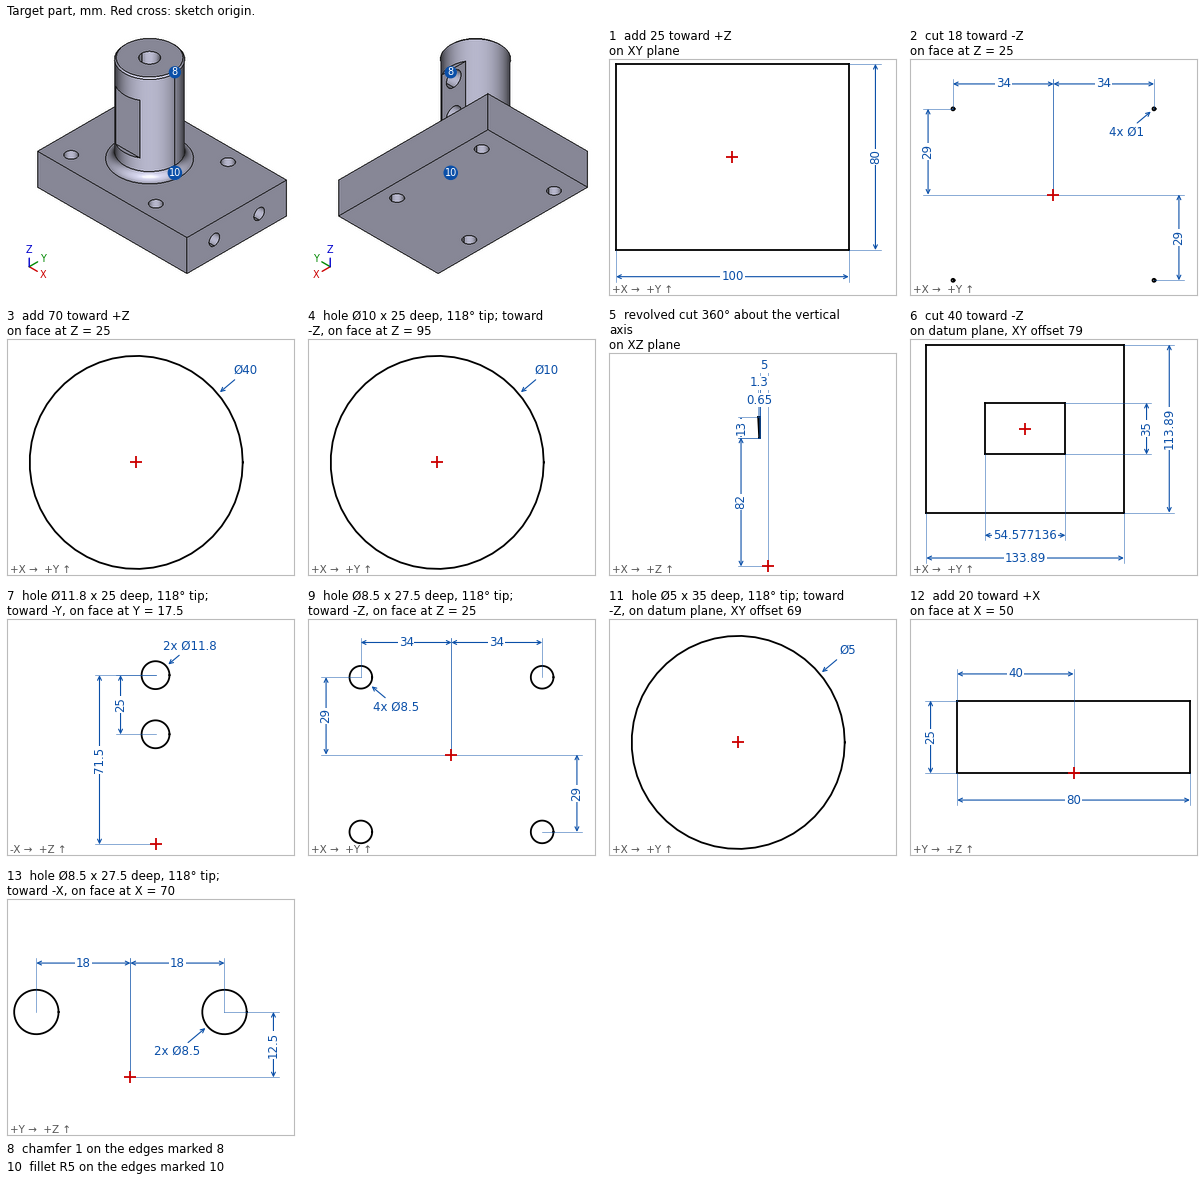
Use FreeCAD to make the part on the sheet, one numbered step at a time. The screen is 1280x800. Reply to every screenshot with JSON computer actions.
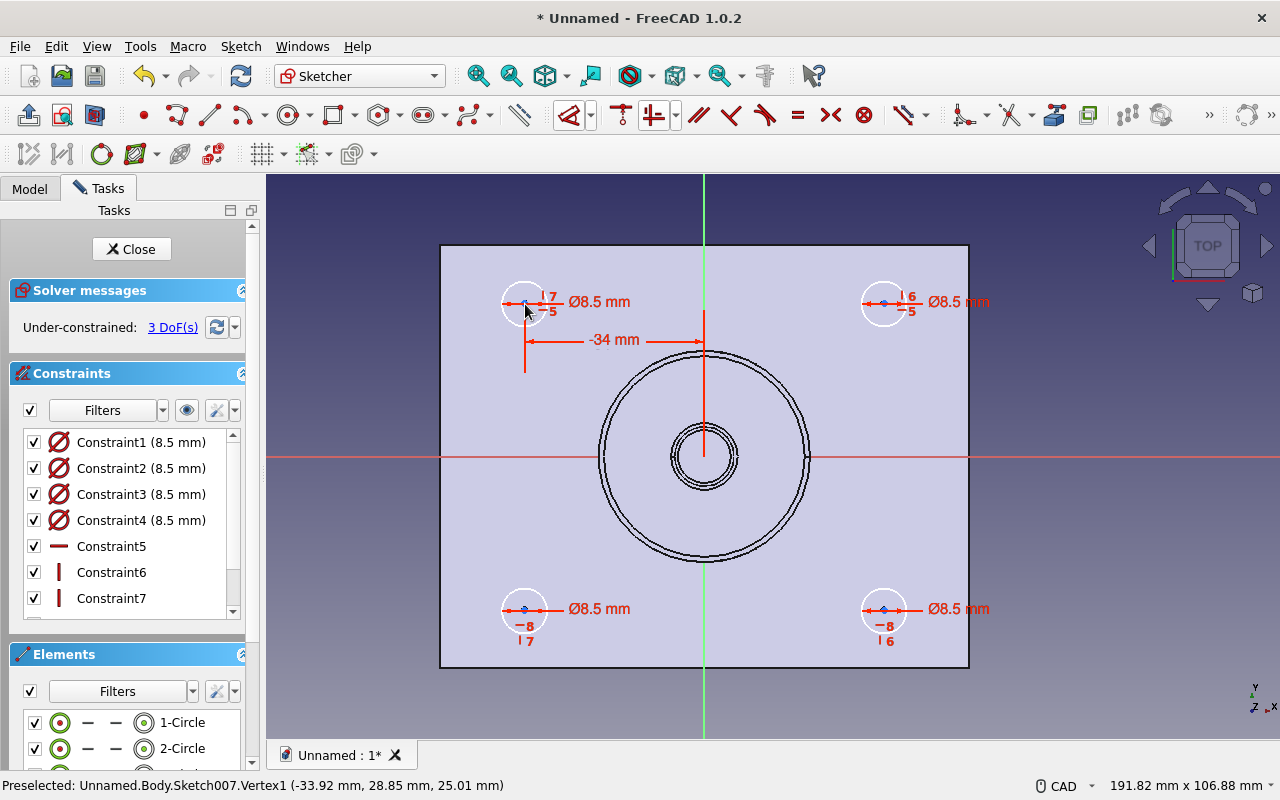
{"action": "left_click", "coordinate": [525, 304]}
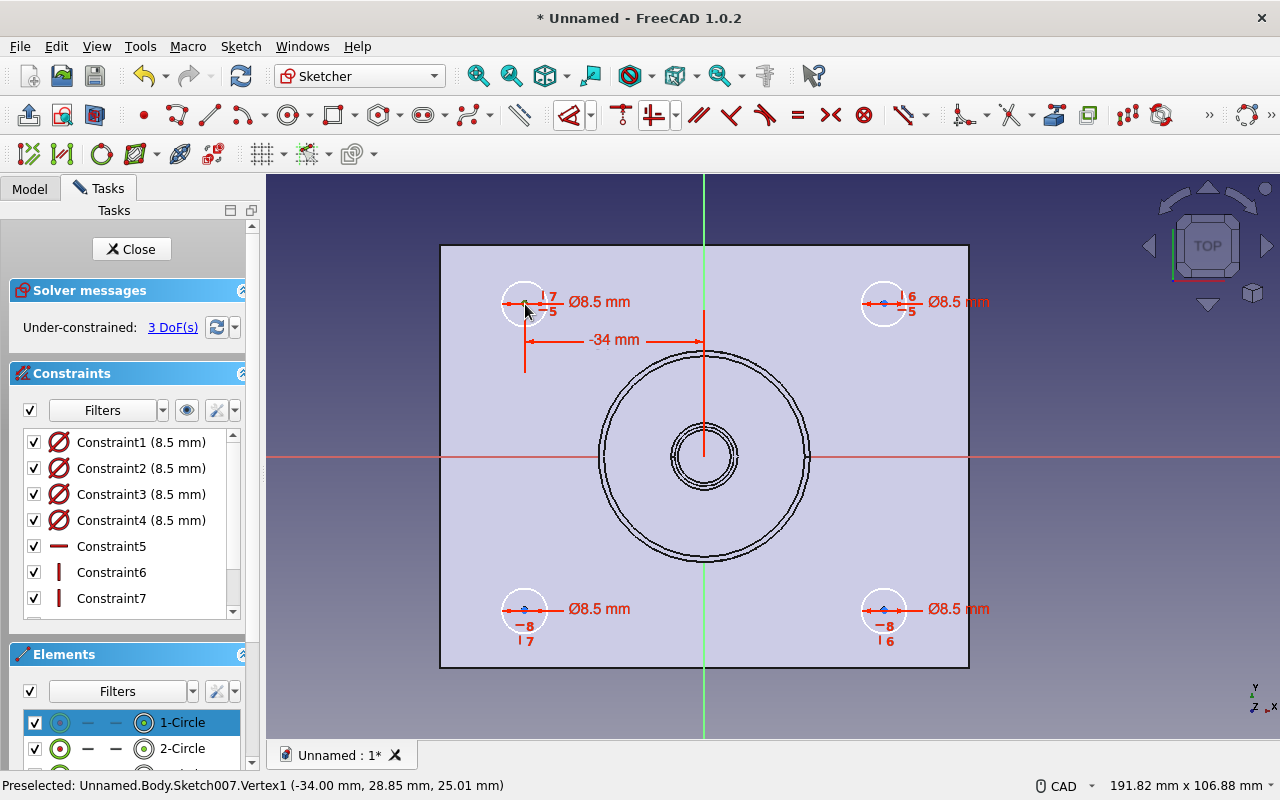
{"action": "key", "text": "i"}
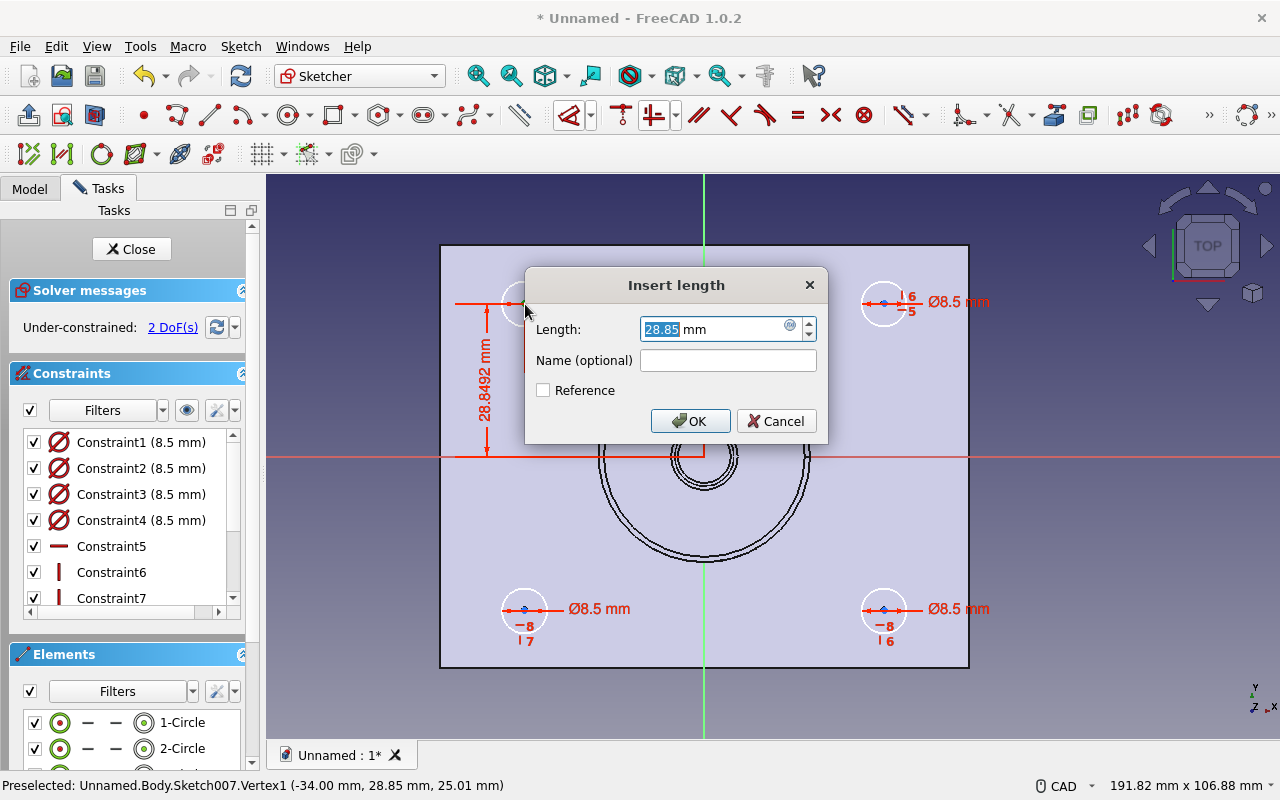
{"action": "type", "text": "29"}
{"action": "key", "text": "Return"}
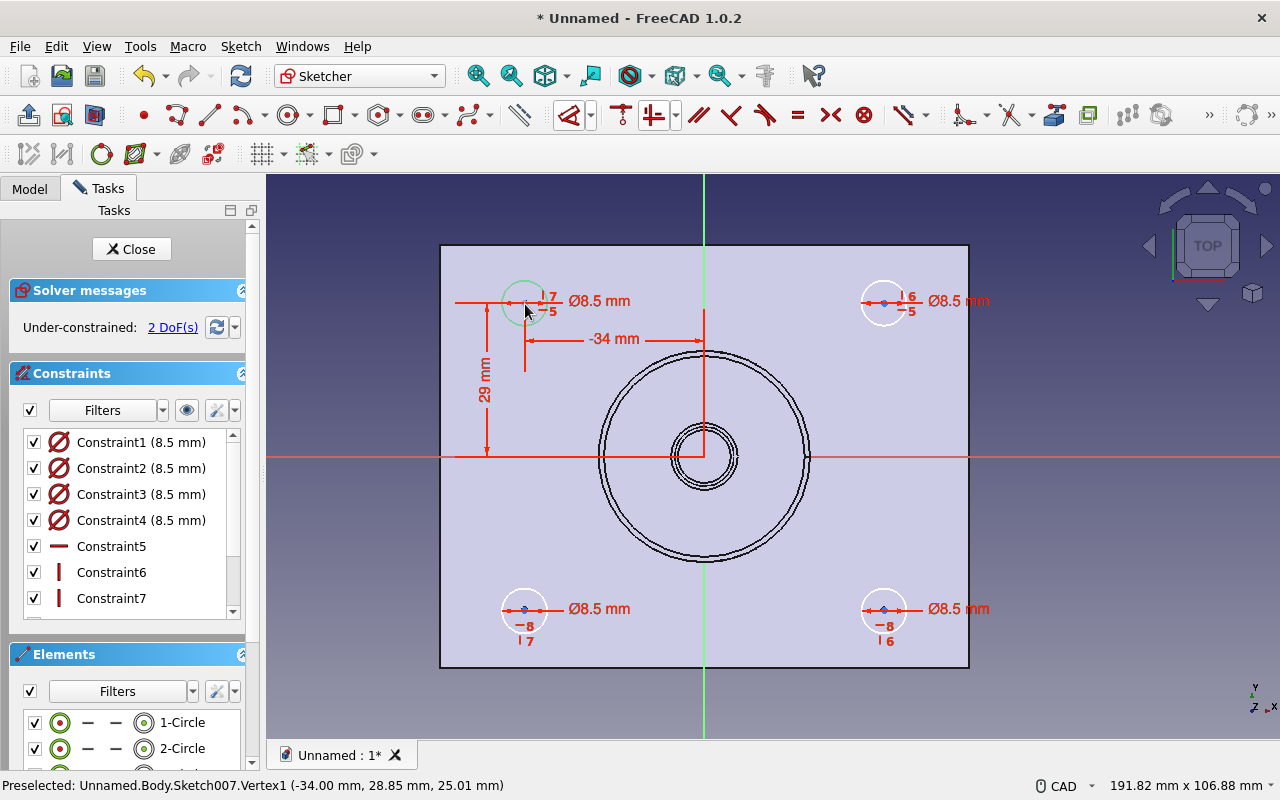
{"action": "left_click", "coordinate": [884, 303]}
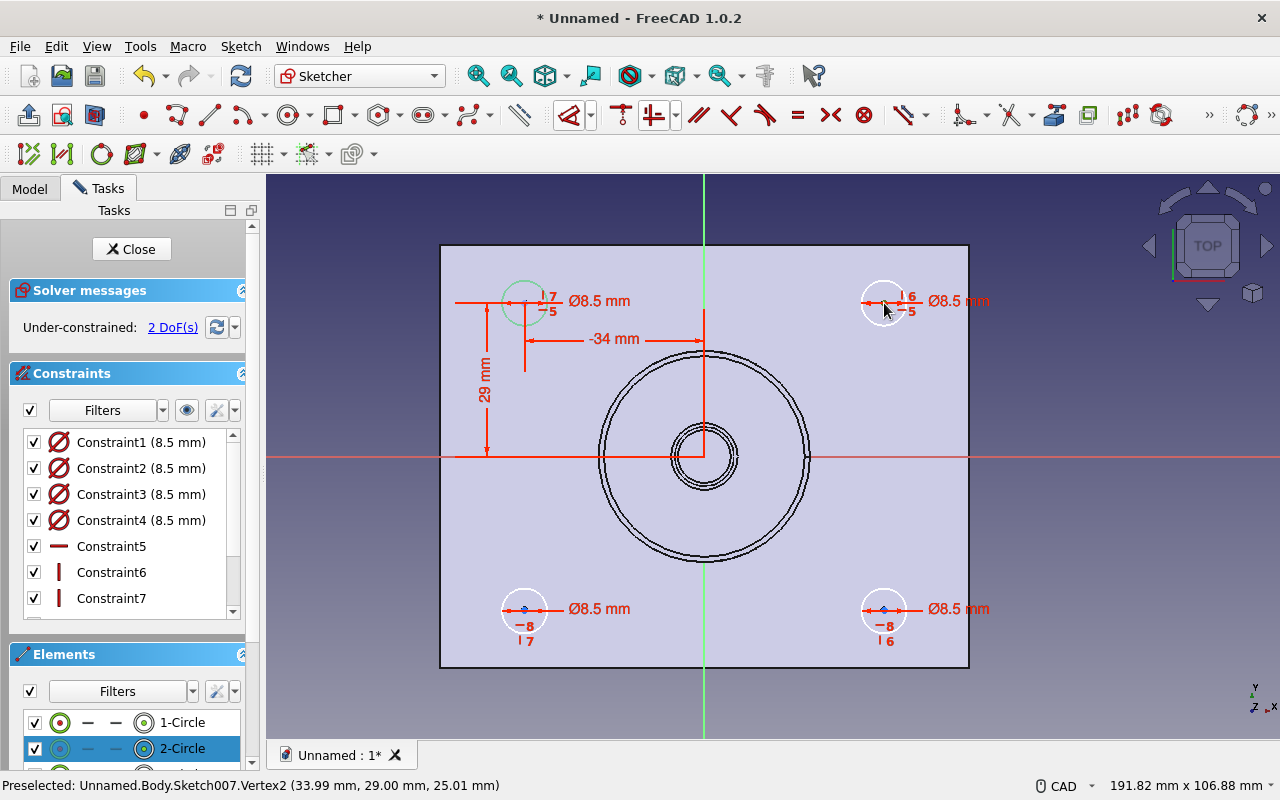
{"action": "key", "text": "l"}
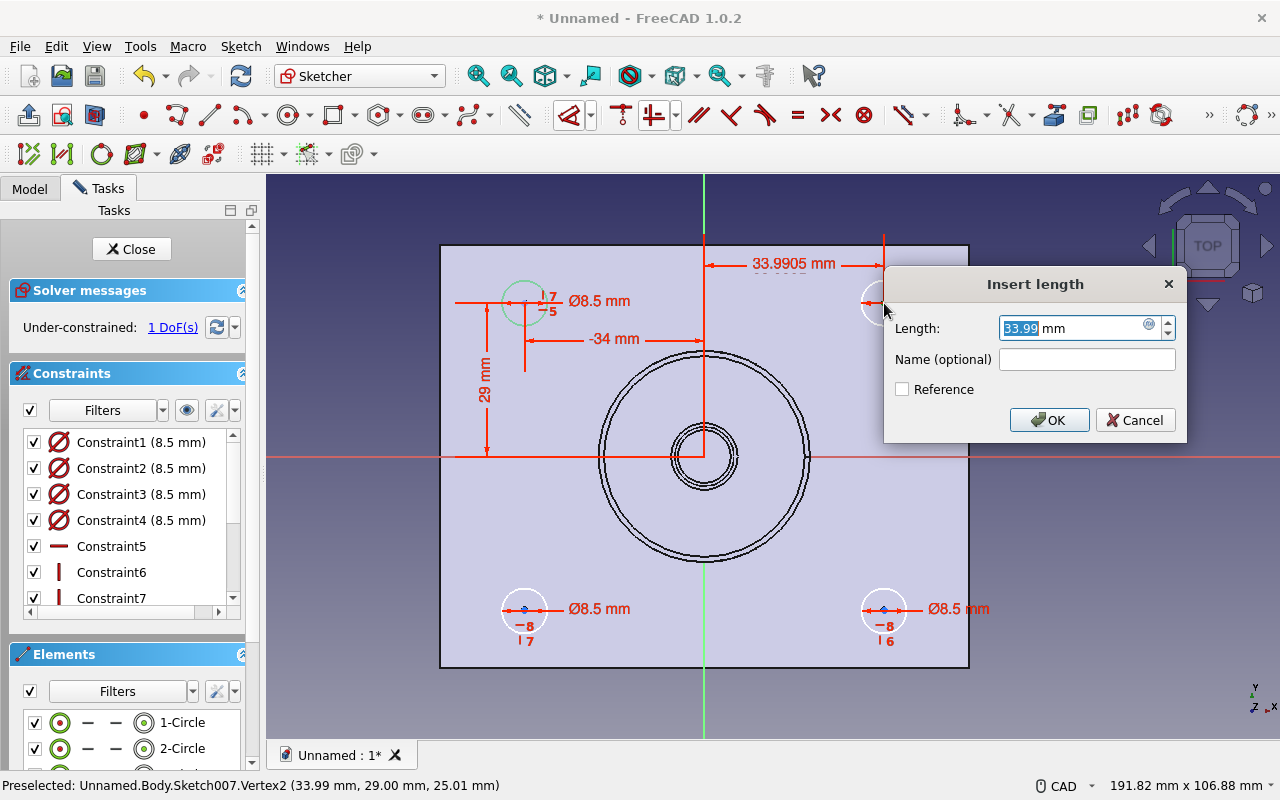
{"action": "type", "text": "34"}
{"action": "key", "text": "Return"}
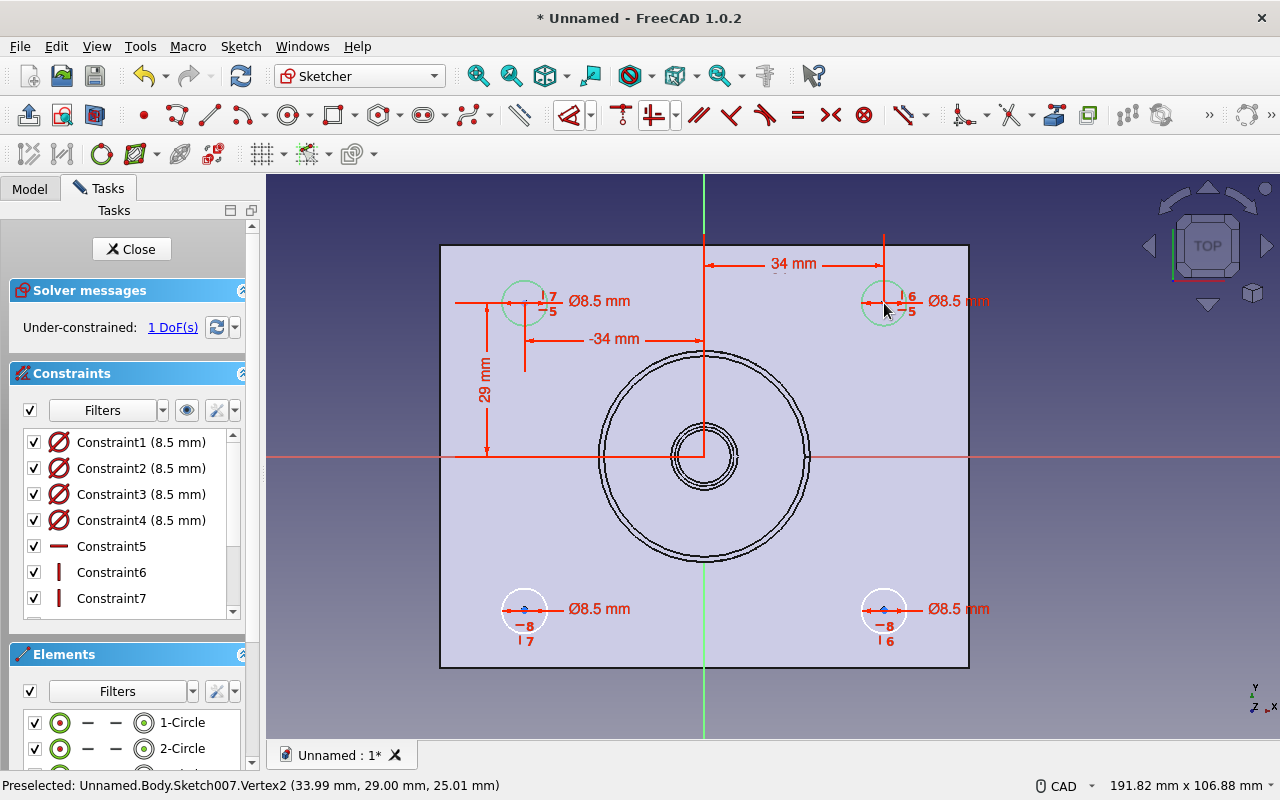
{"action": "left_click", "coordinate": [884, 611]}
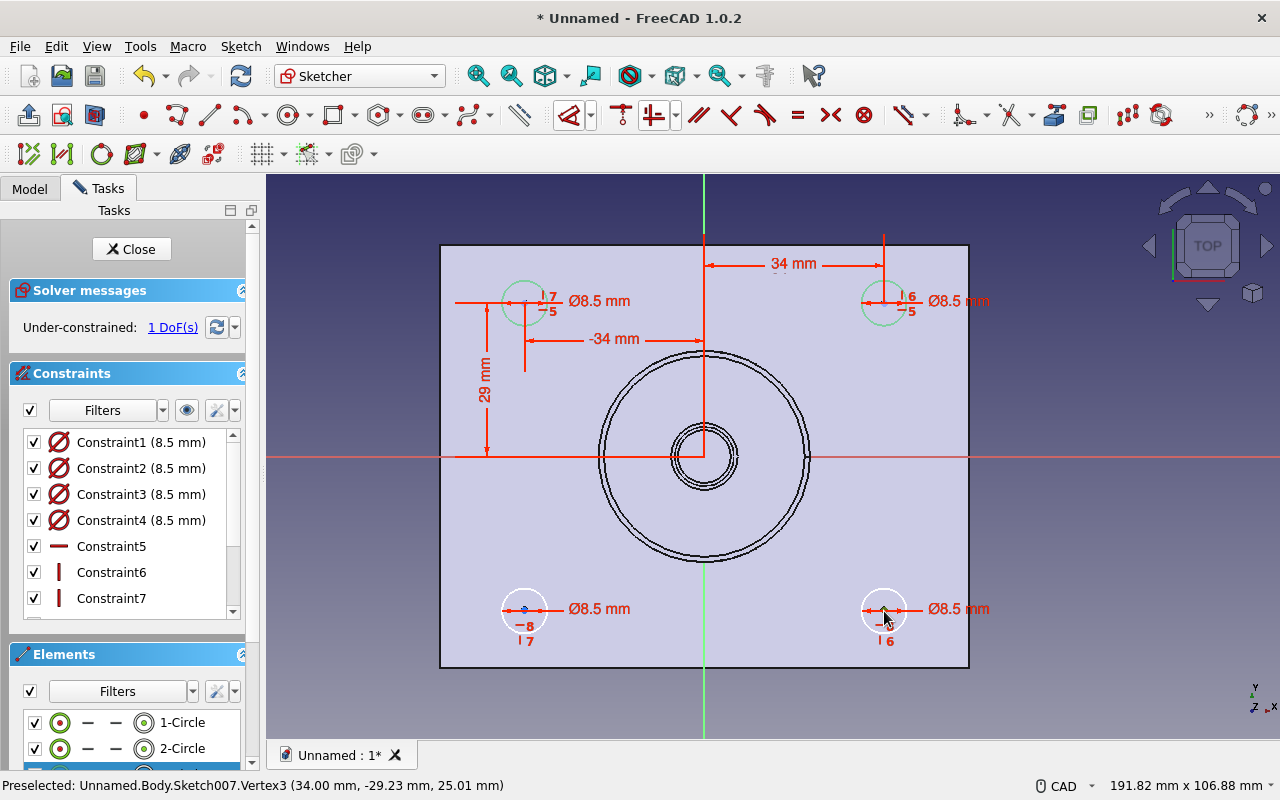
{"action": "left_click", "coordinate": [590, 116]}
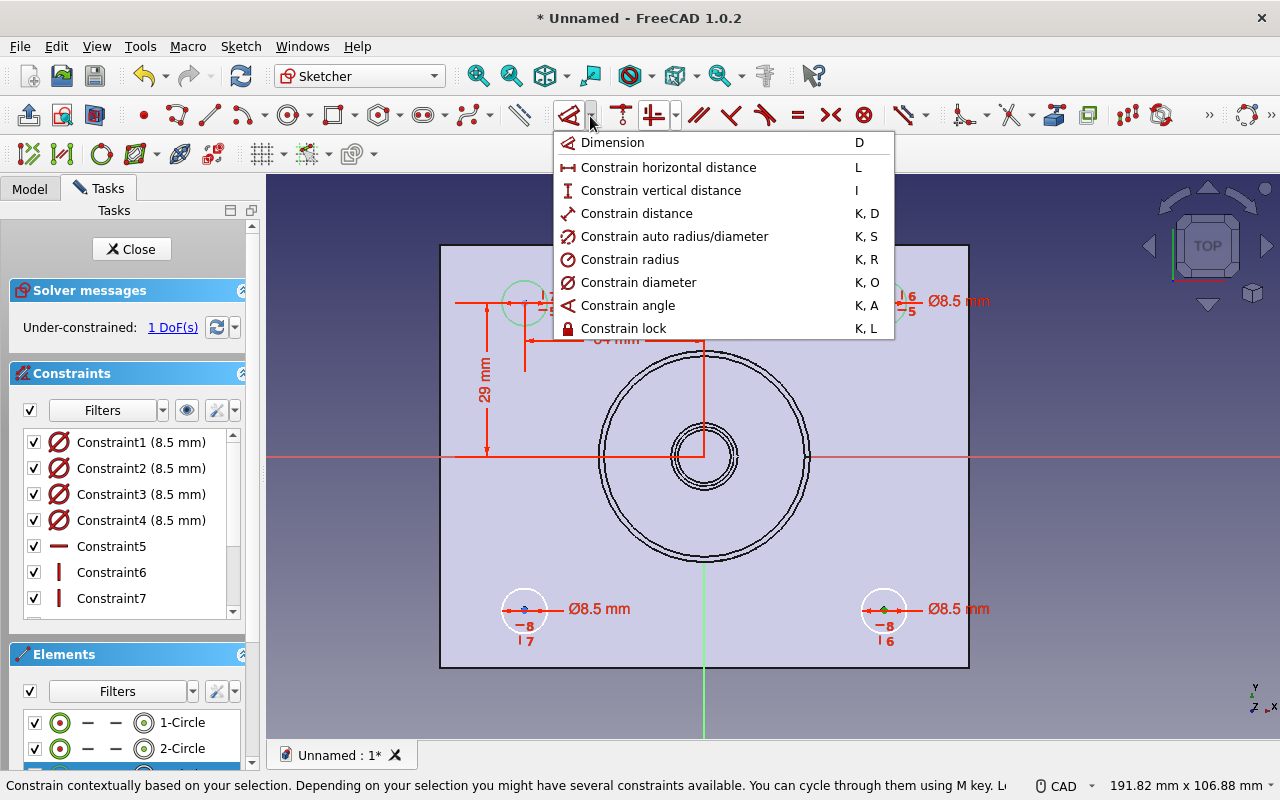
{"action": "left_click", "coordinate": [724, 190]}